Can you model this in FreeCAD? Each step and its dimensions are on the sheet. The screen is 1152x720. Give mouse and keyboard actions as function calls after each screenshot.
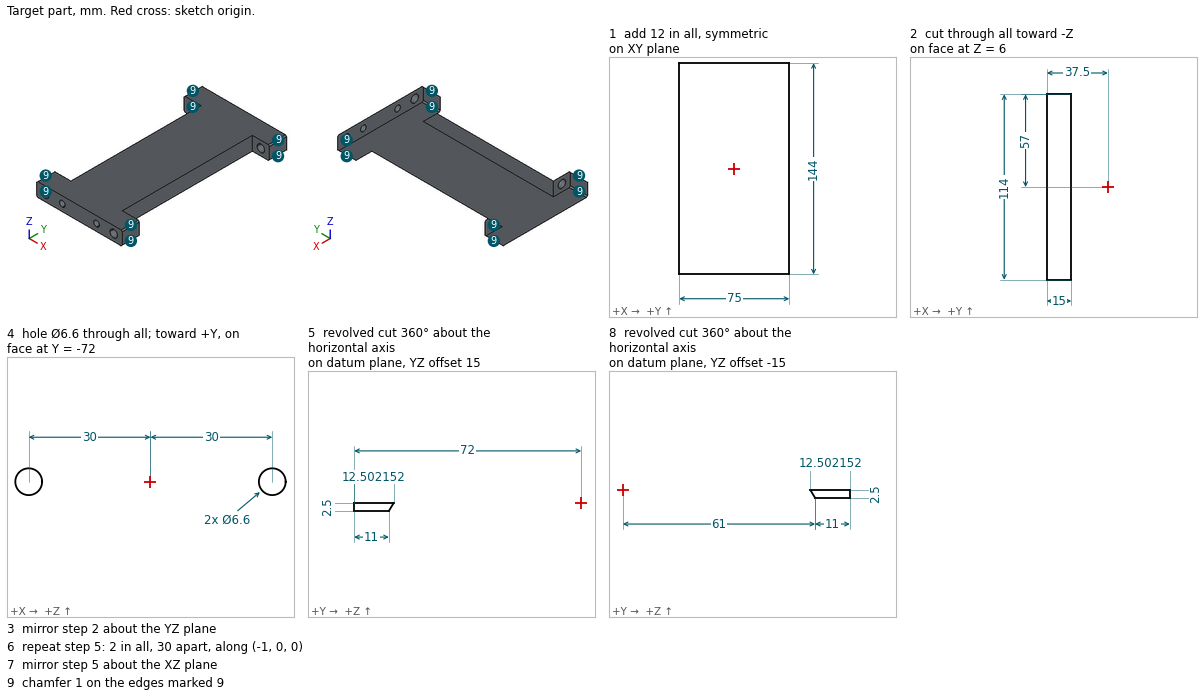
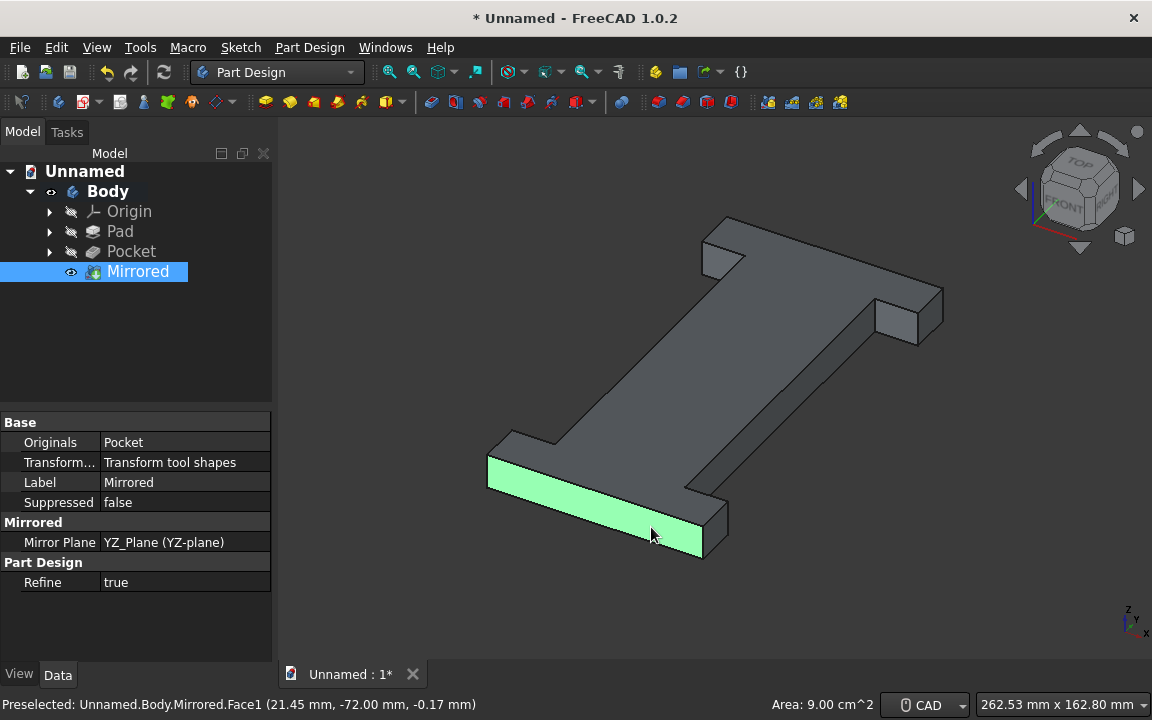
click(84, 102)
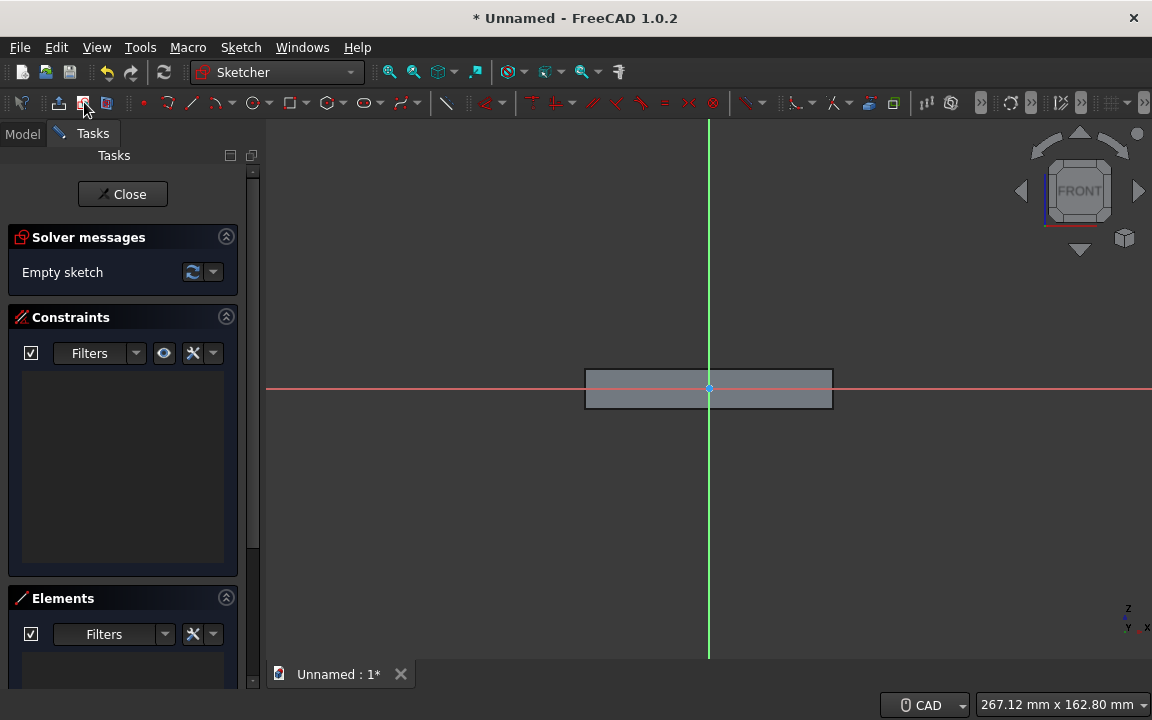
scroll(765, 389, up, 4)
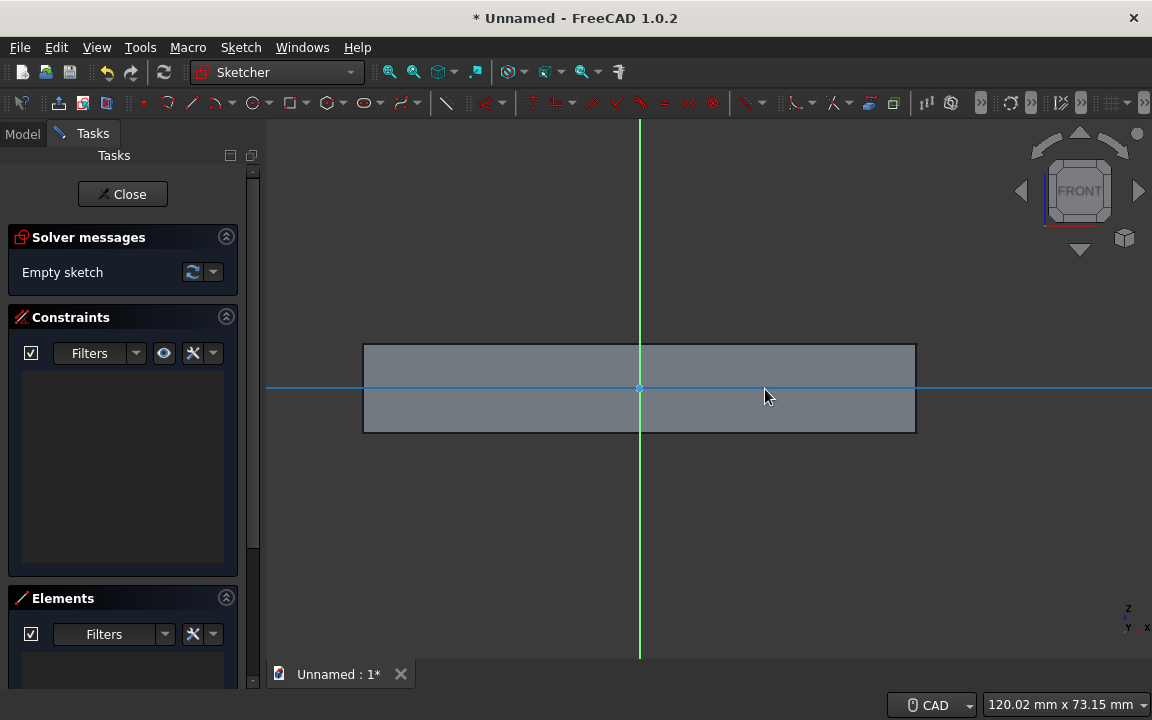
click(254, 104)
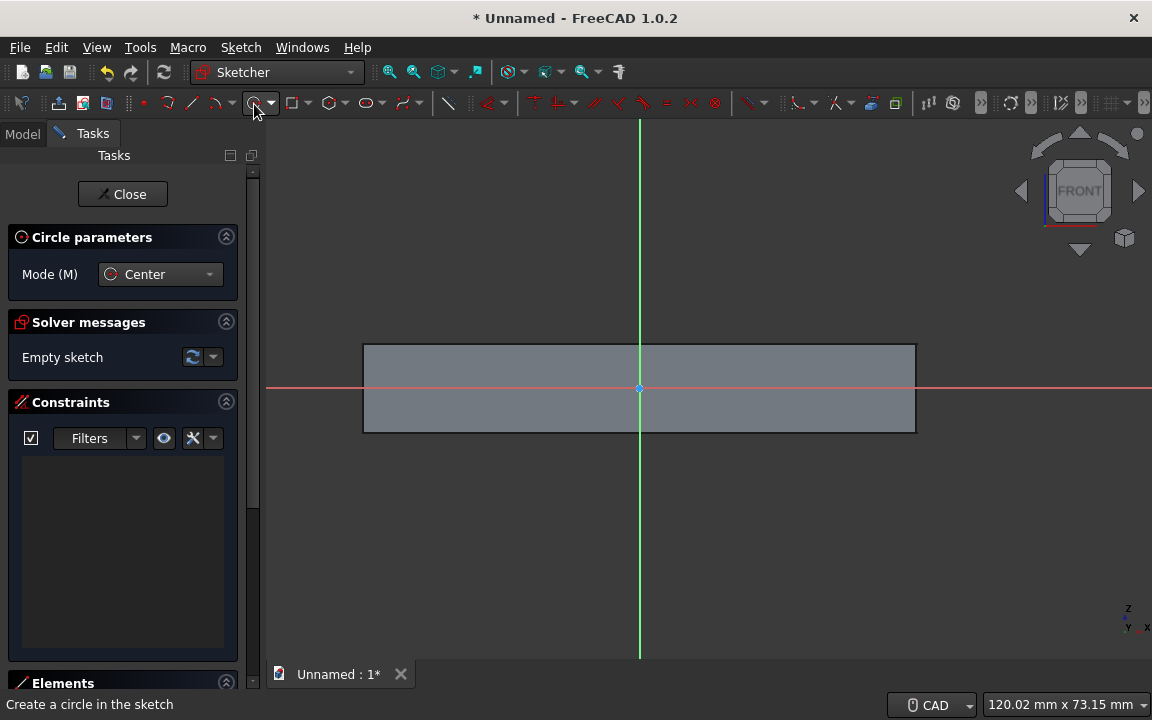
click(861, 388)
move(878, 371)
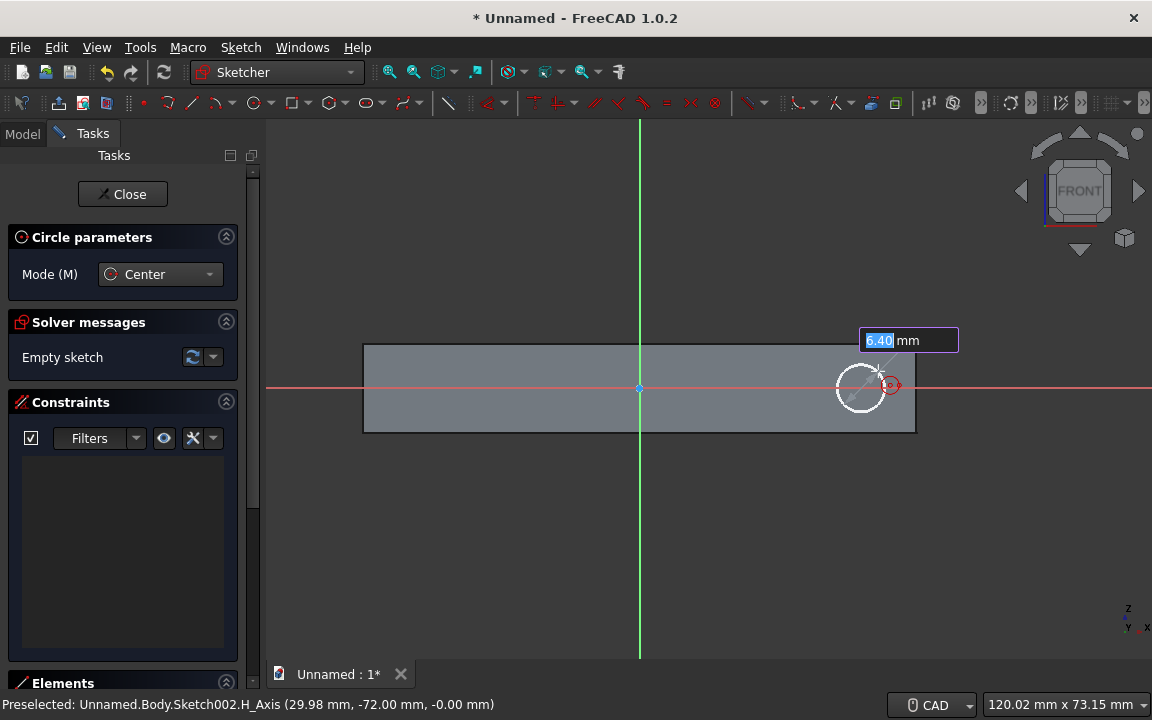
text(6.6)
key(Return)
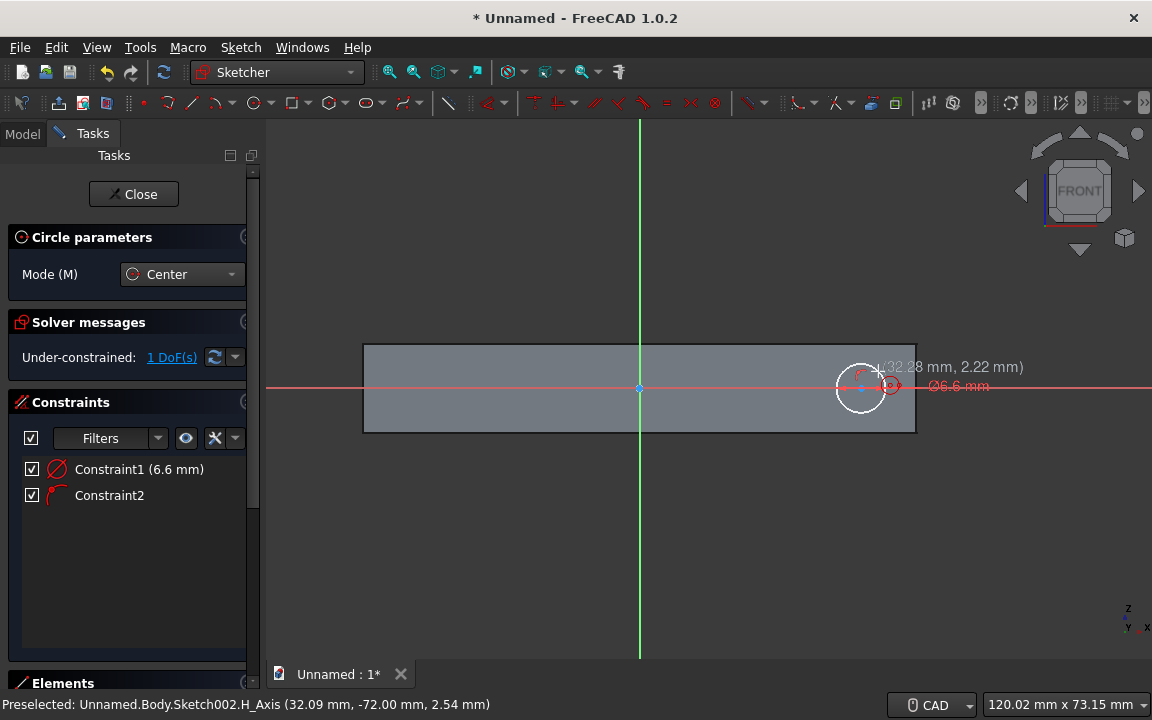
click(418, 388)
move(435, 371)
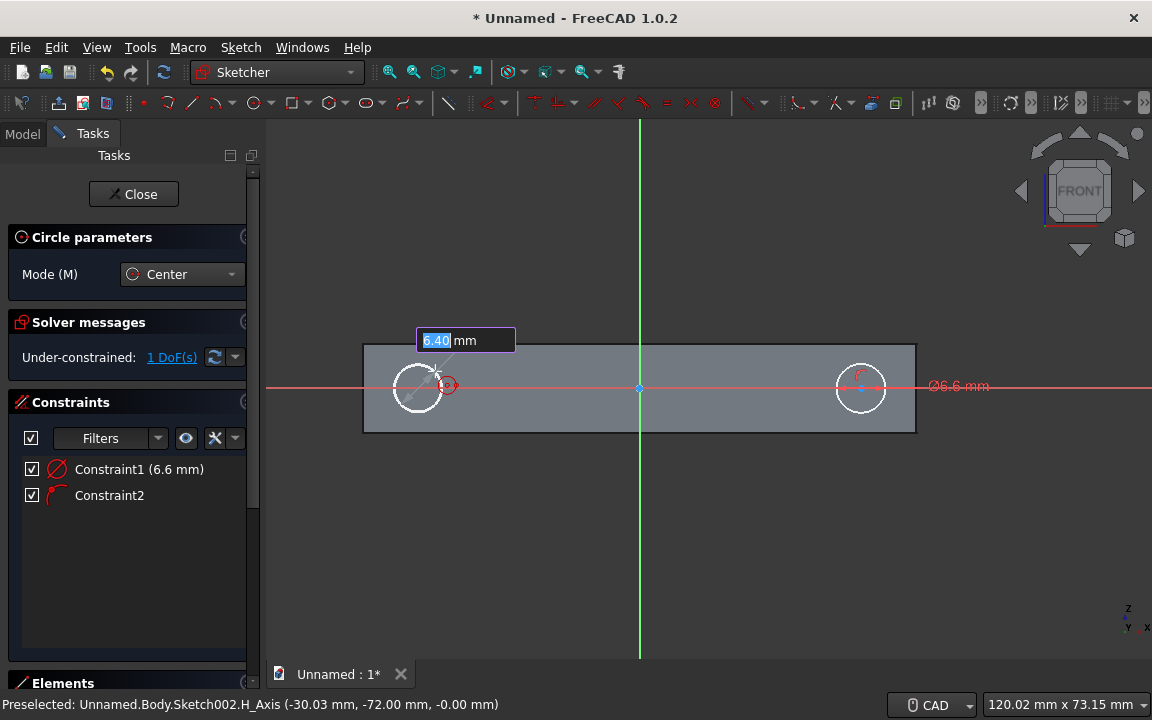
text(6.6)
key(Return)
key(Escape)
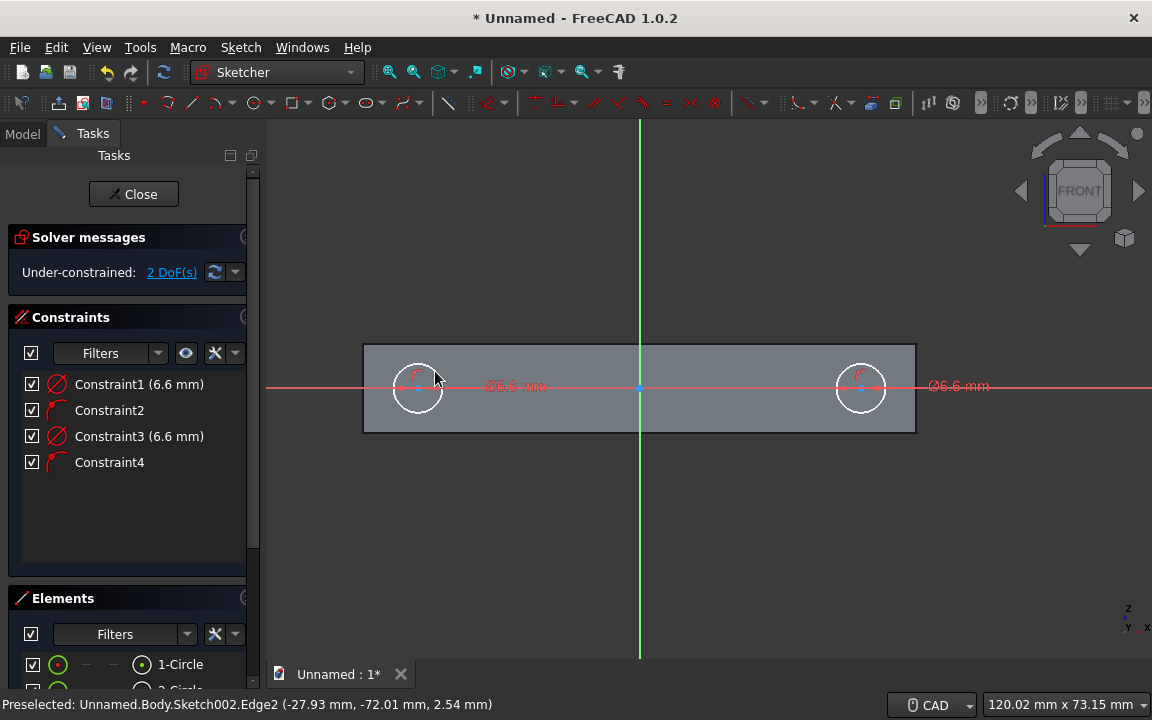
click(488, 104)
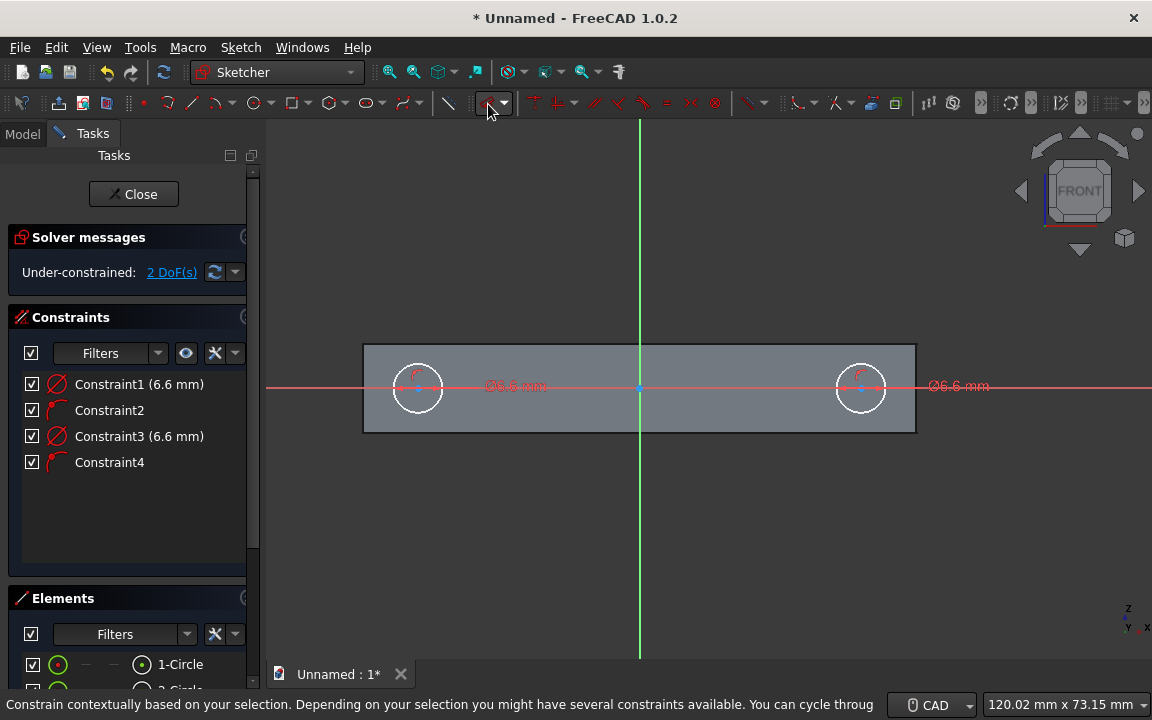
click(861, 388)
click(750, 422)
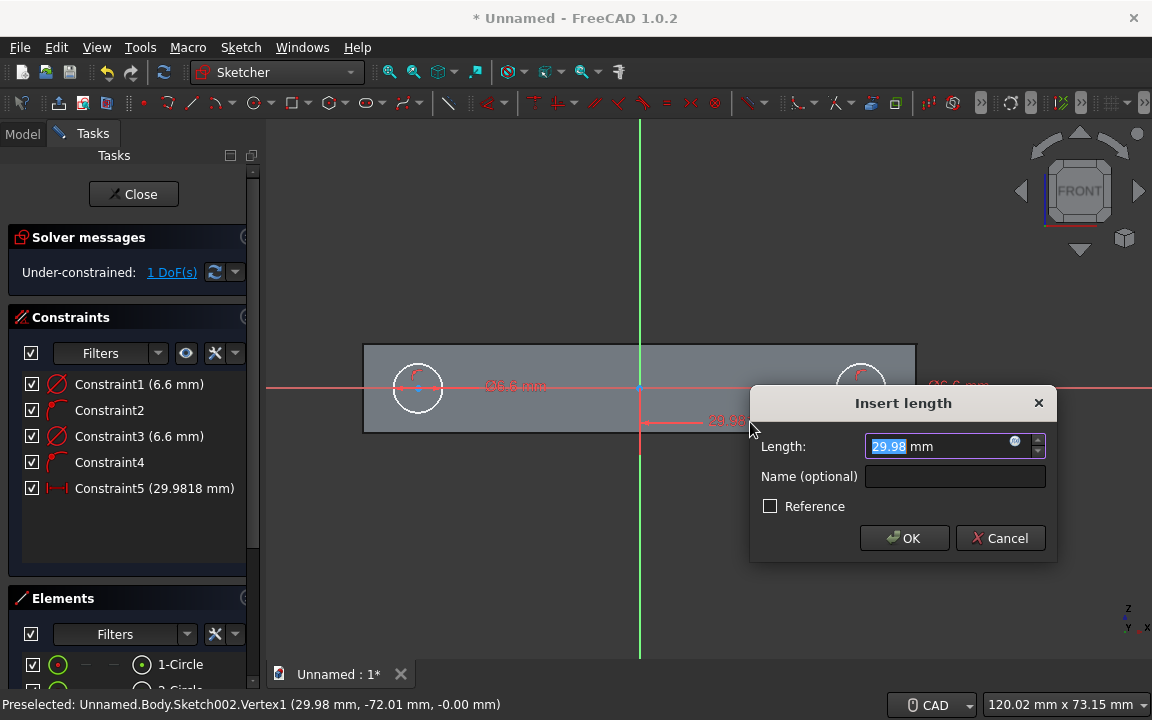
text(30)
key(Return)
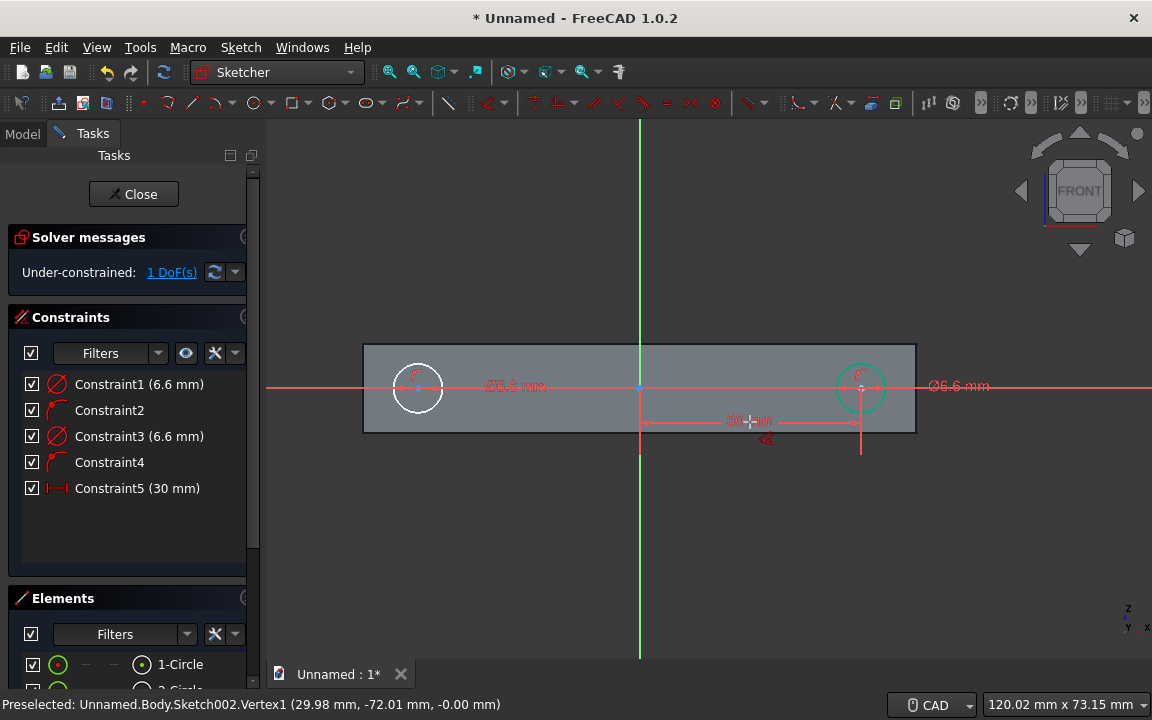
click(418, 388)
click(529, 422)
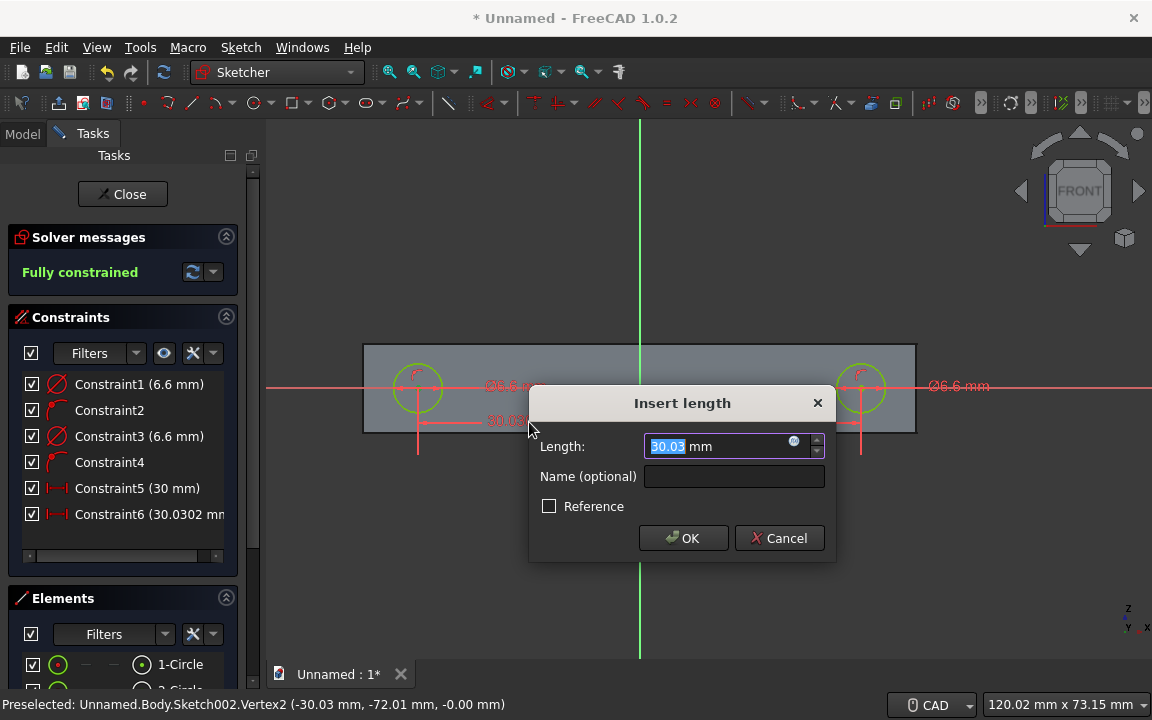
text(30)
key(Return)
key(Escape)